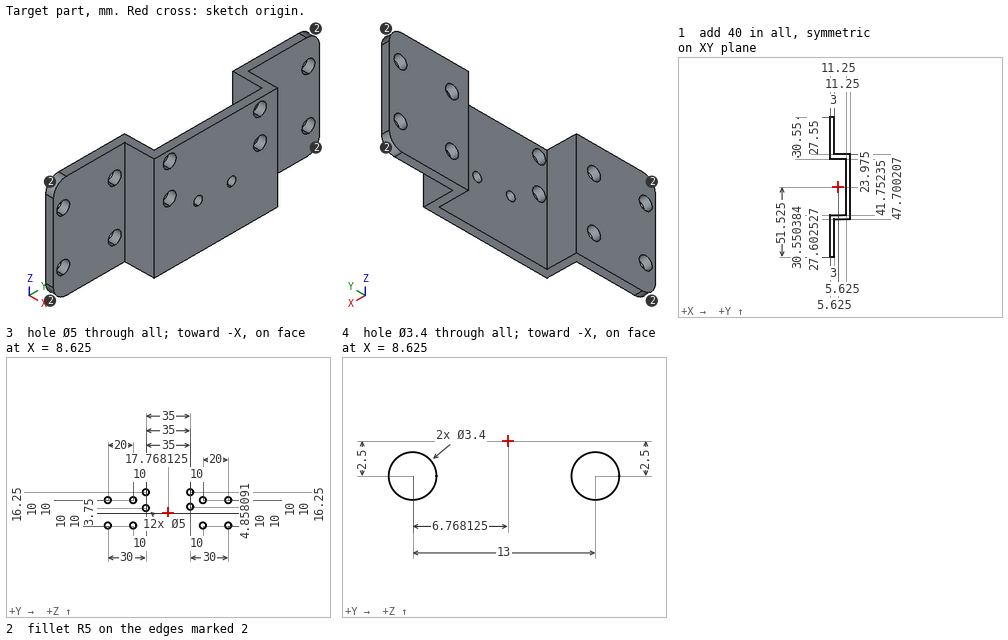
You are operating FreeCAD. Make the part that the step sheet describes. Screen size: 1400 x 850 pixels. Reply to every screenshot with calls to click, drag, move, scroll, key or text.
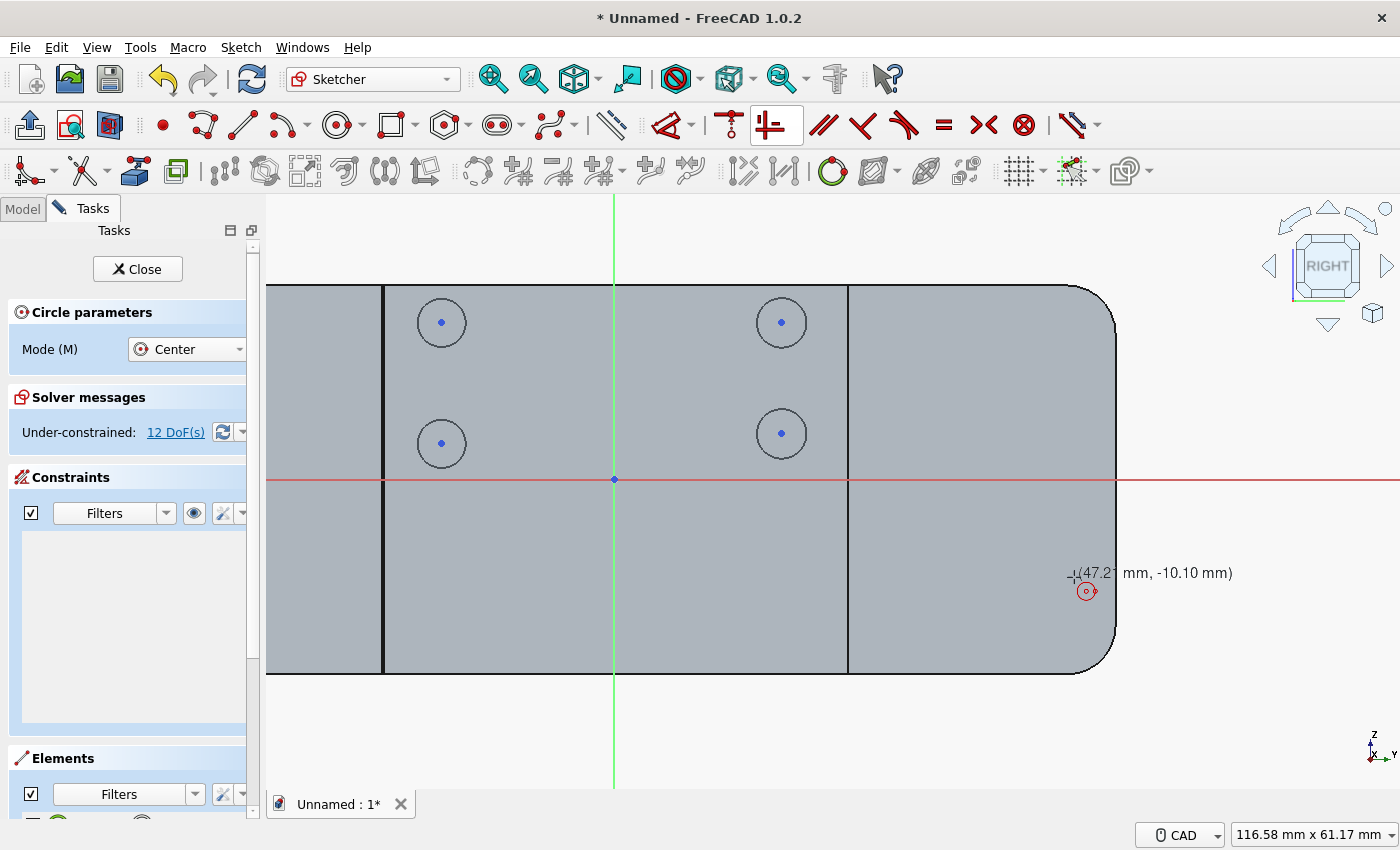
click(1074, 577)
click(1091, 560)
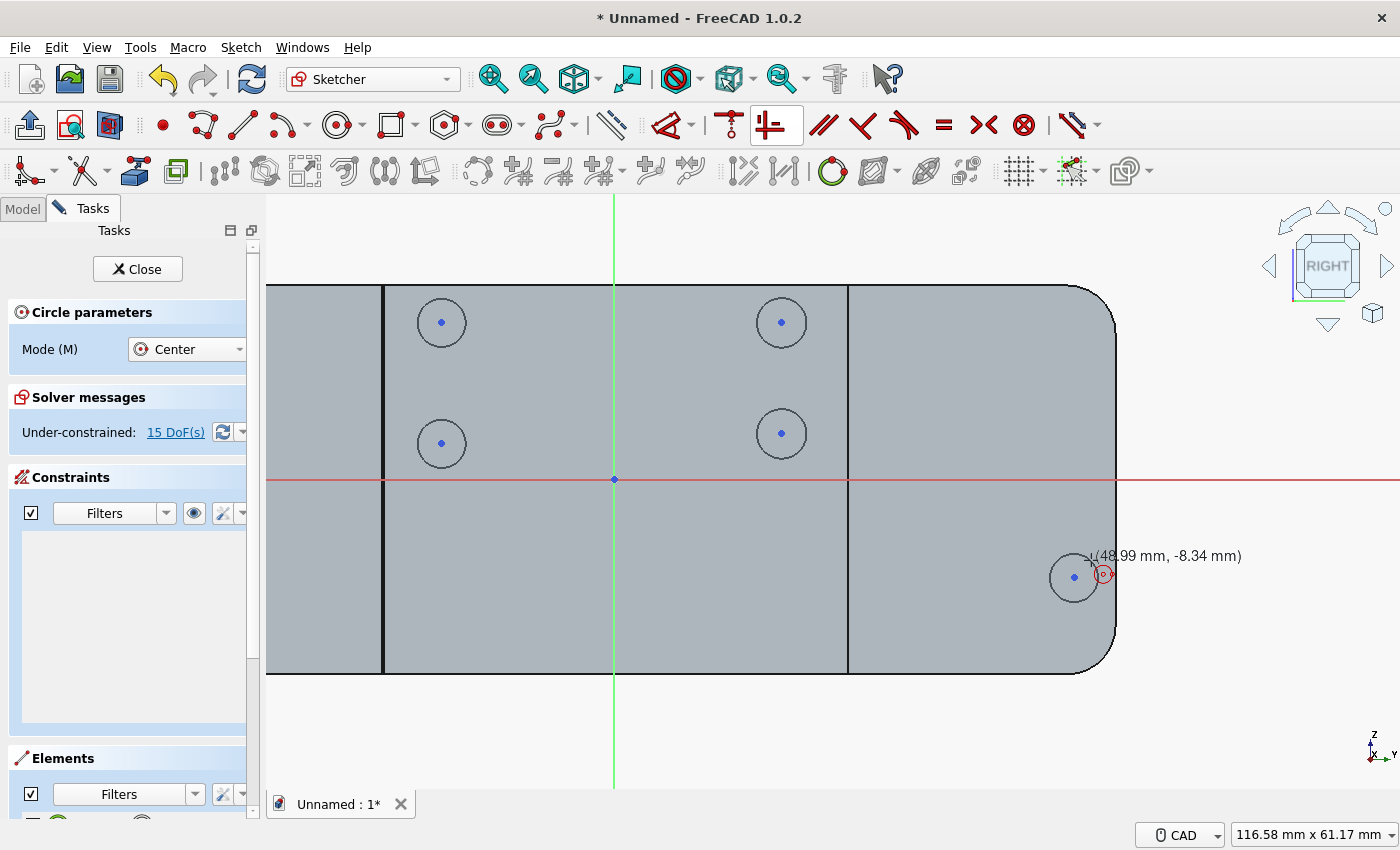
click(879, 577)
click(897, 560)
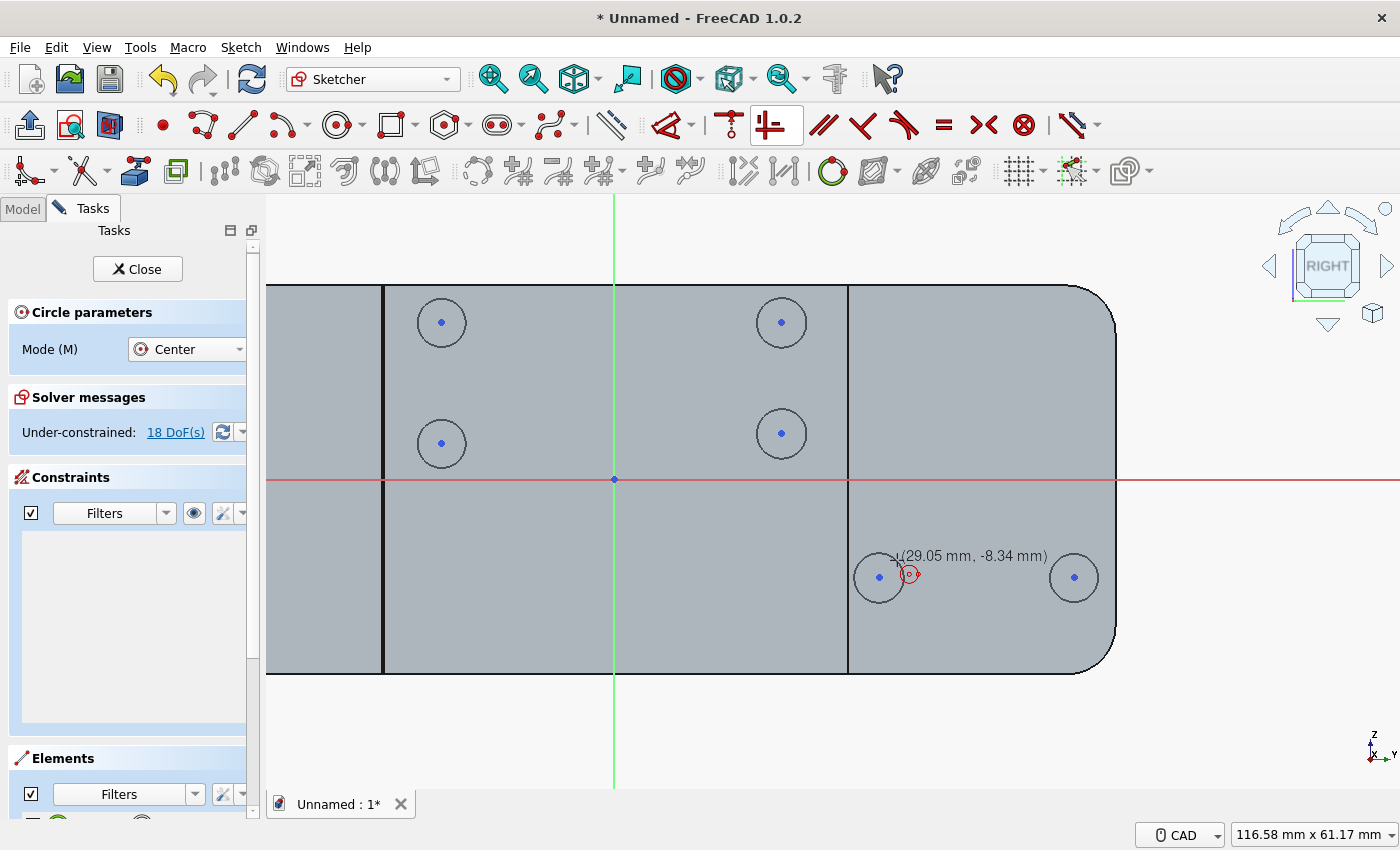
click(879, 383)
click(897, 365)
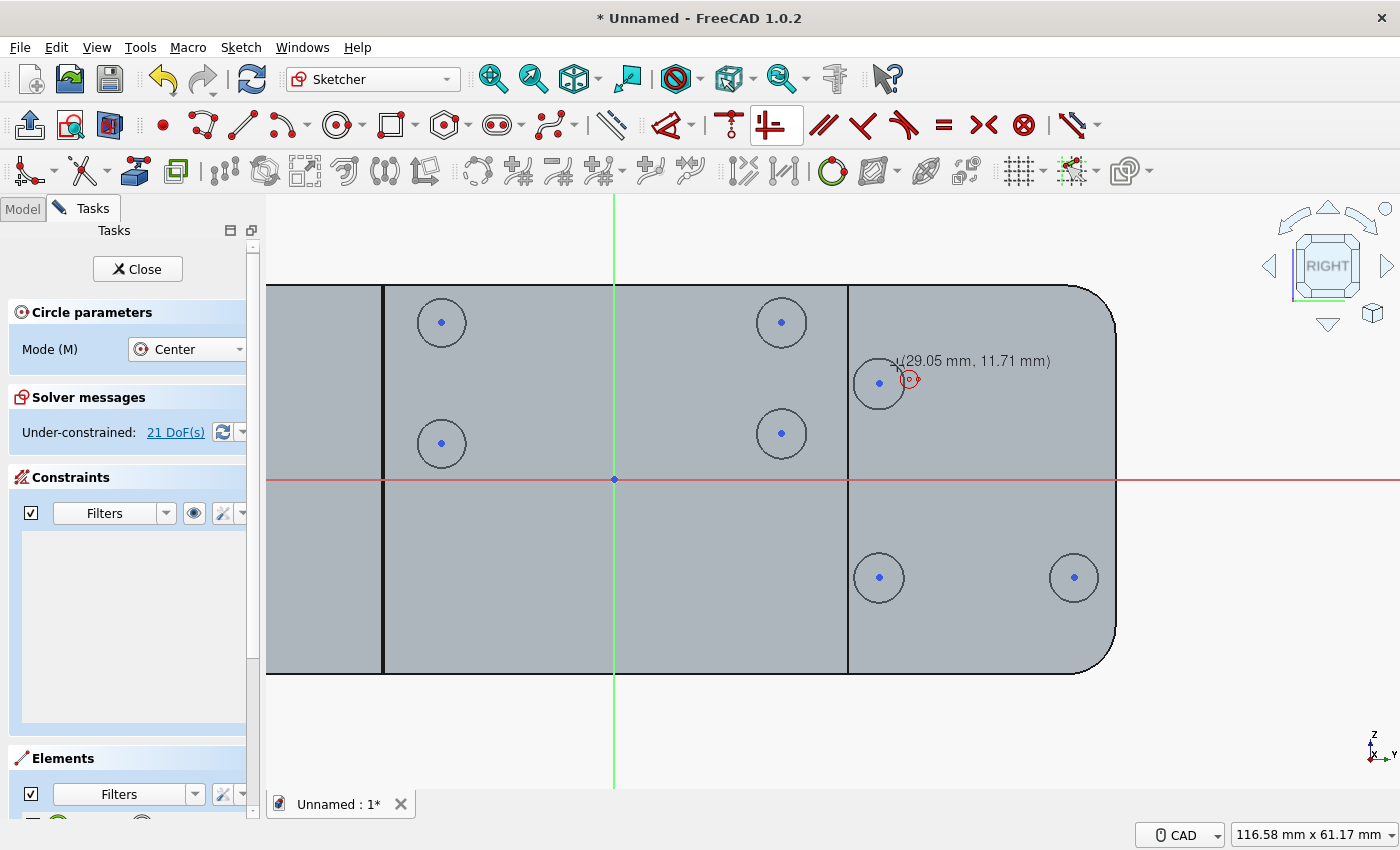
click(1074, 383)
click(1091, 365)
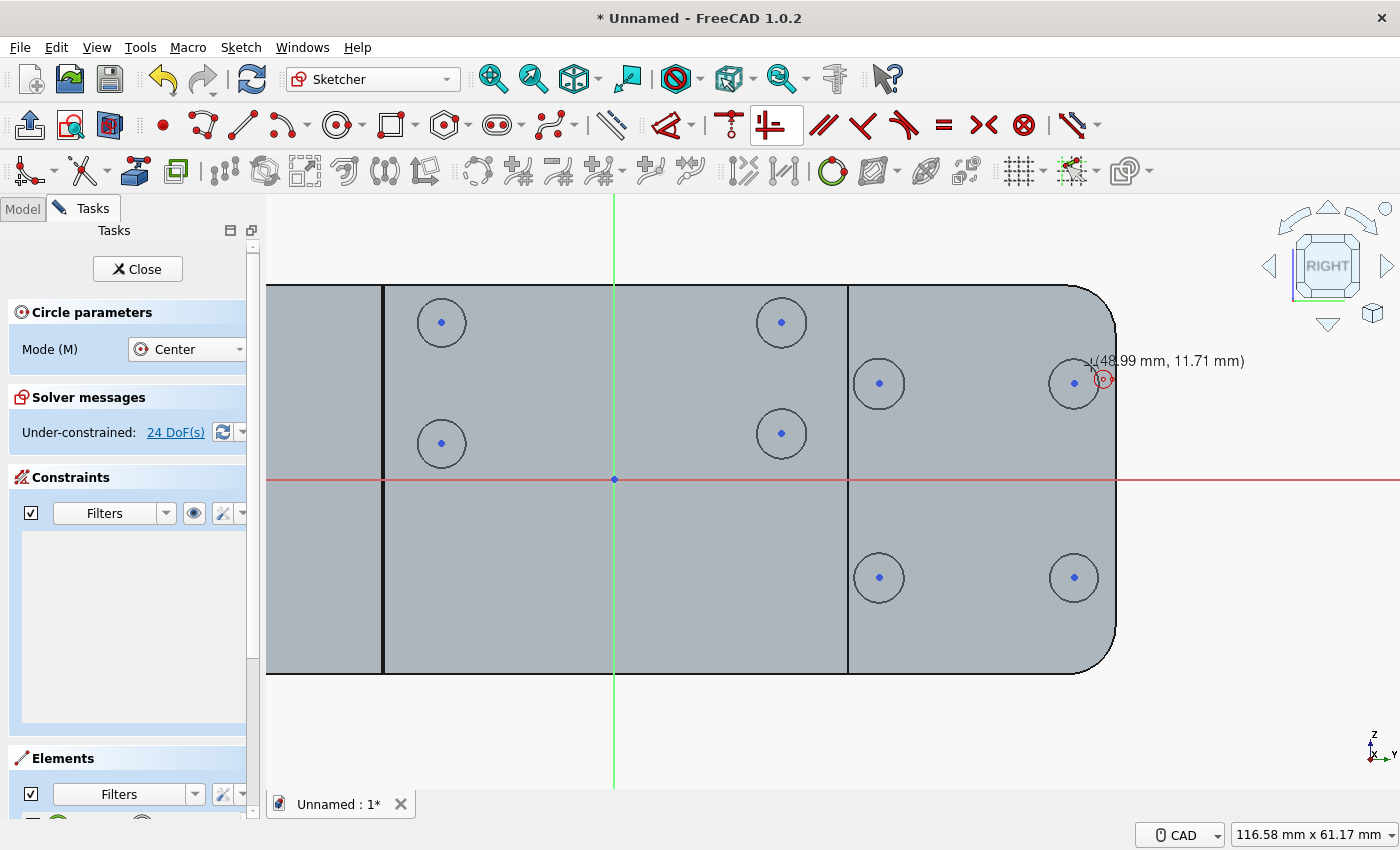
scroll(1075, 577, down, 2)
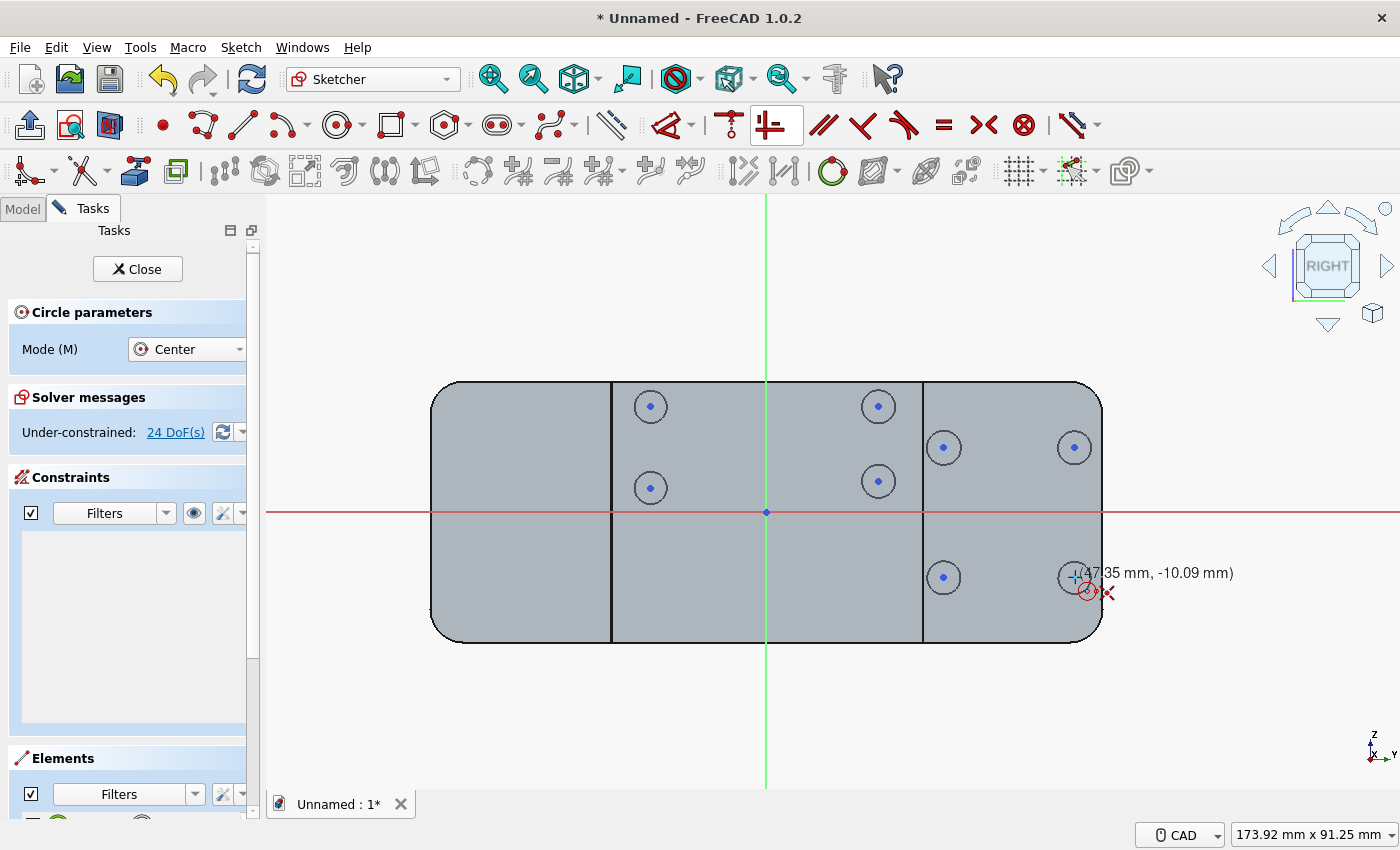
scroll(455, 577, up, 2)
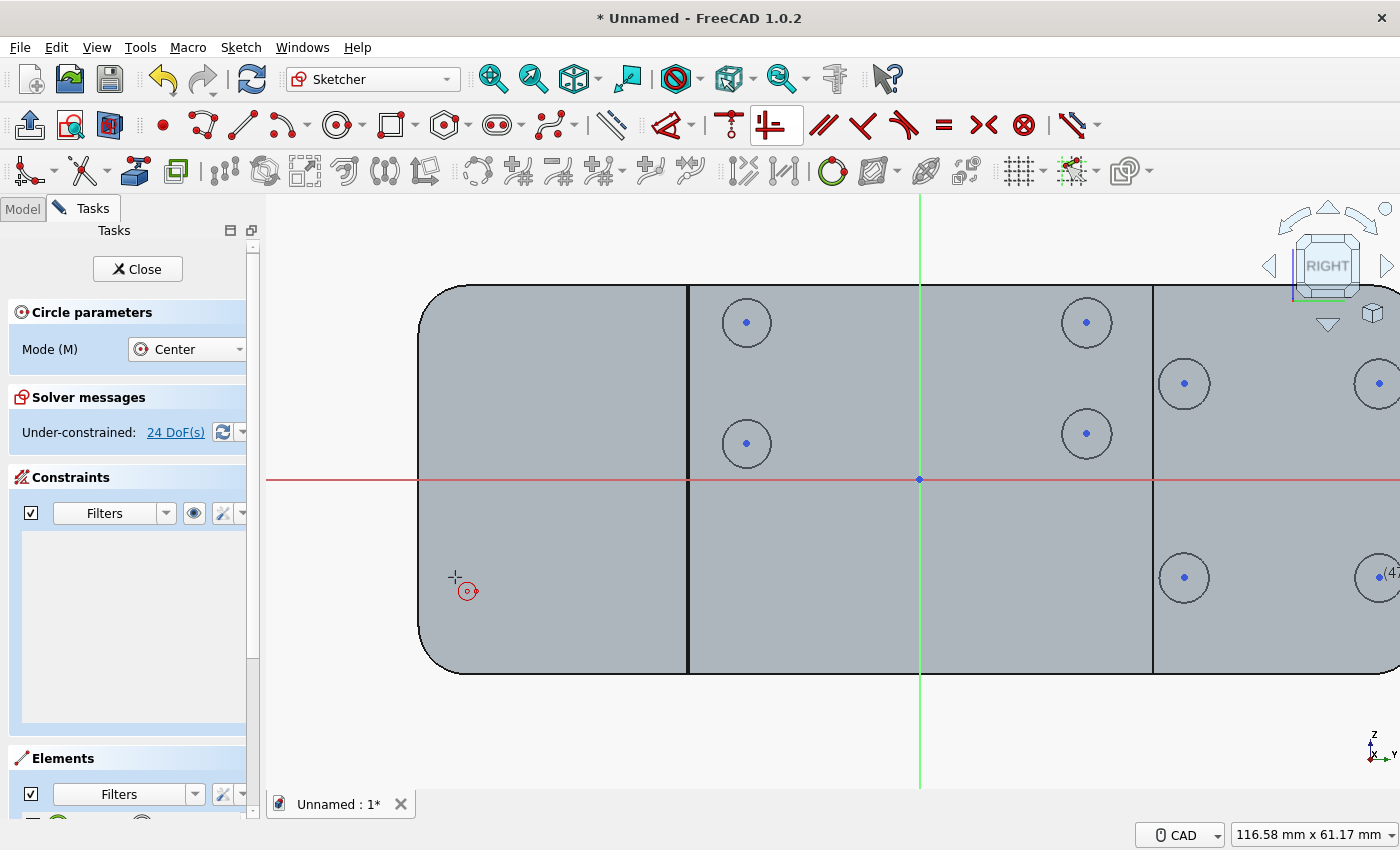
click(455, 577)
click(472, 560)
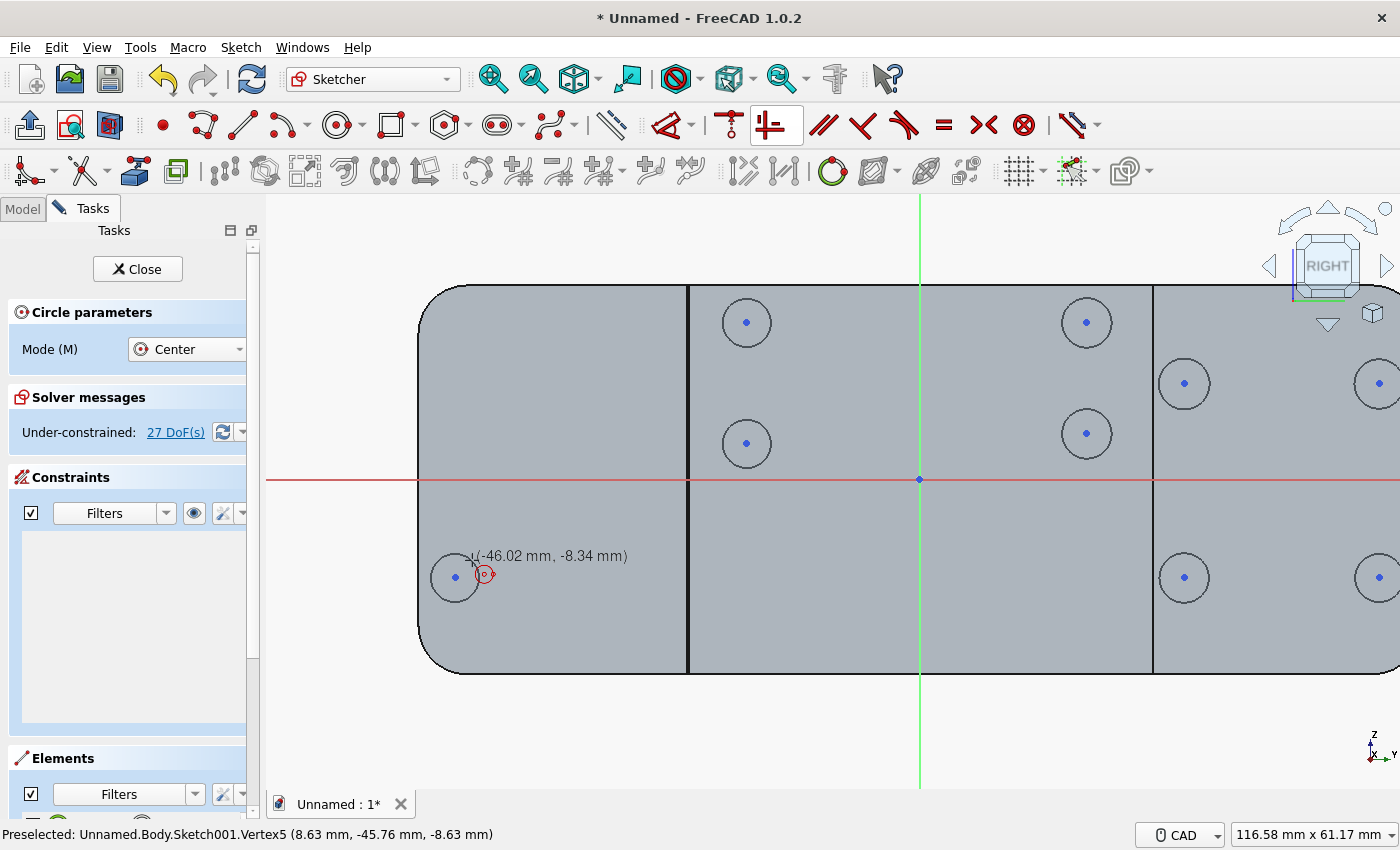
click(650, 577)
click(667, 560)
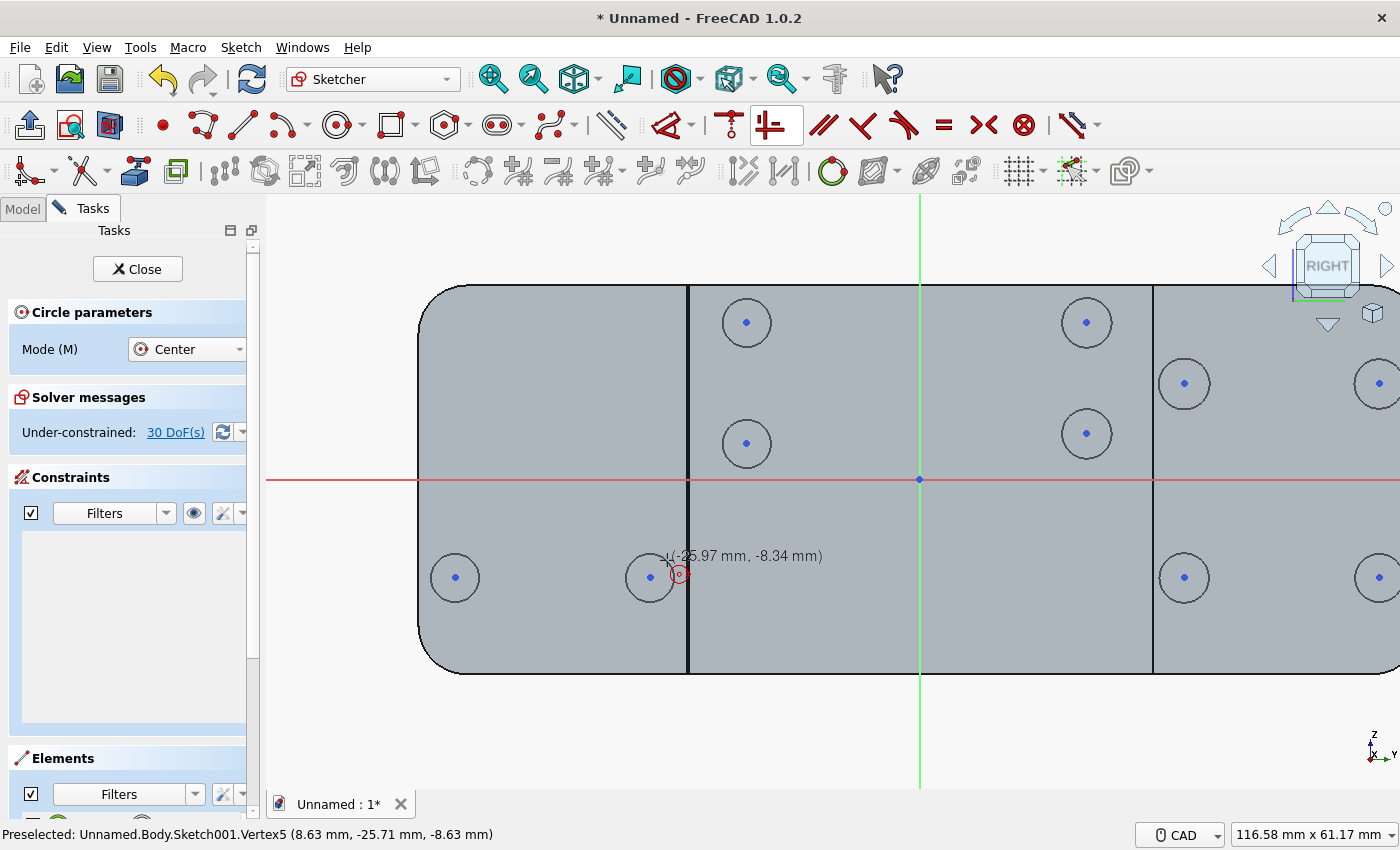
click(650, 383)
click(667, 365)